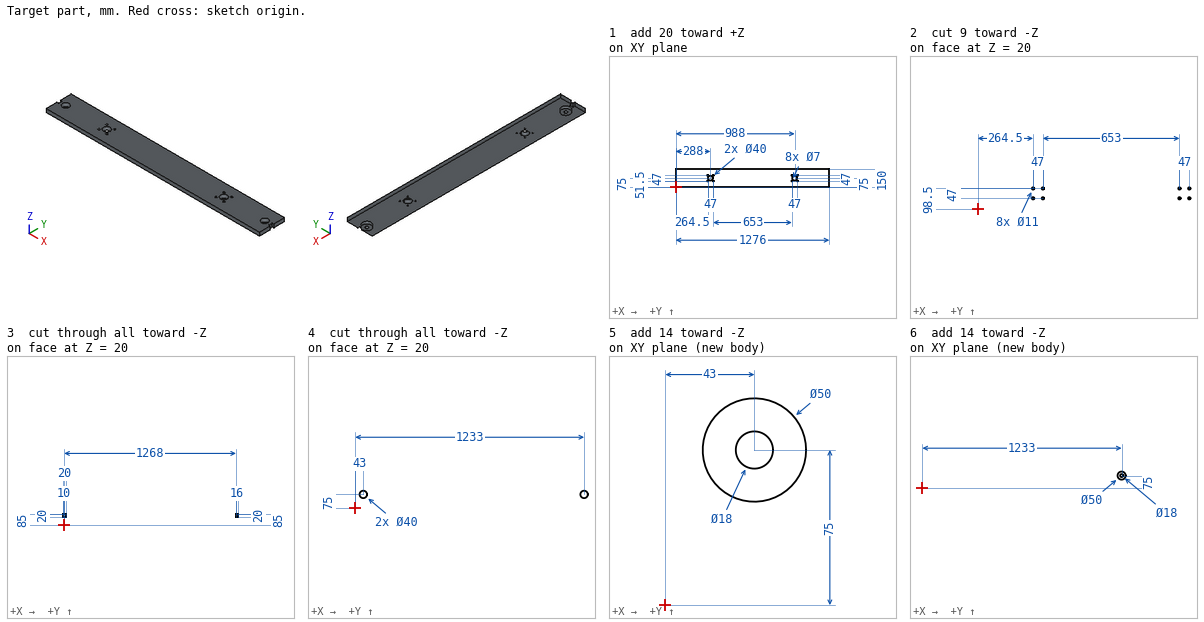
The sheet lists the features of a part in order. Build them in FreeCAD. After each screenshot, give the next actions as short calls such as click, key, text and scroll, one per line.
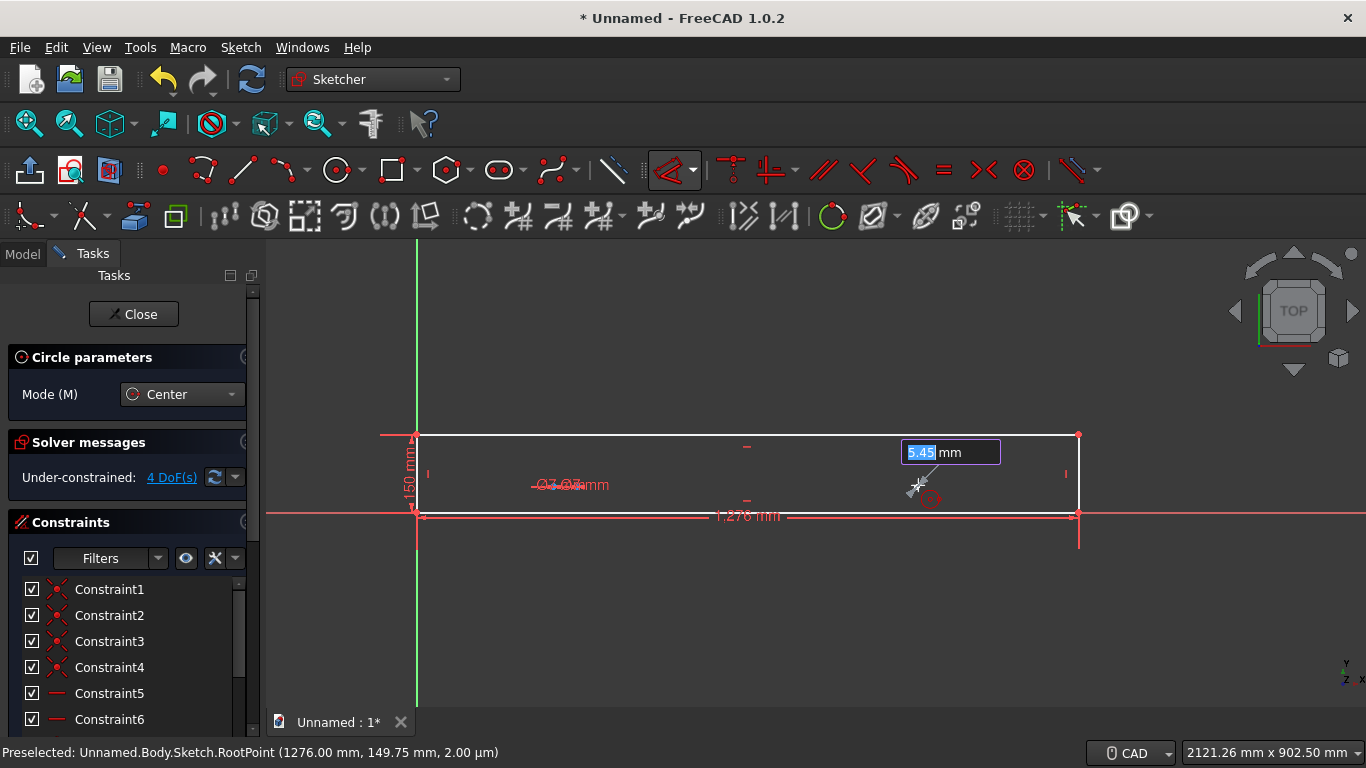
text(7)
key(Return)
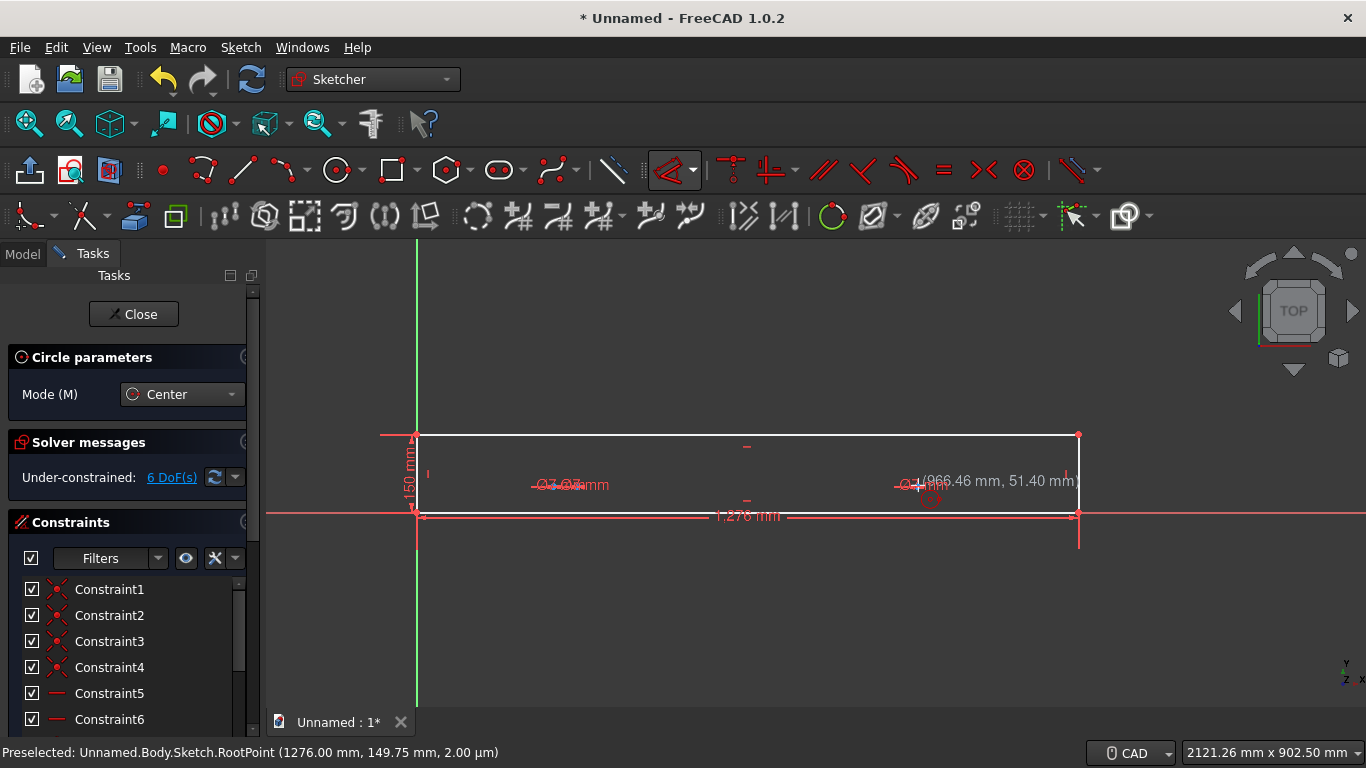
scroll(941, 486, up, 13)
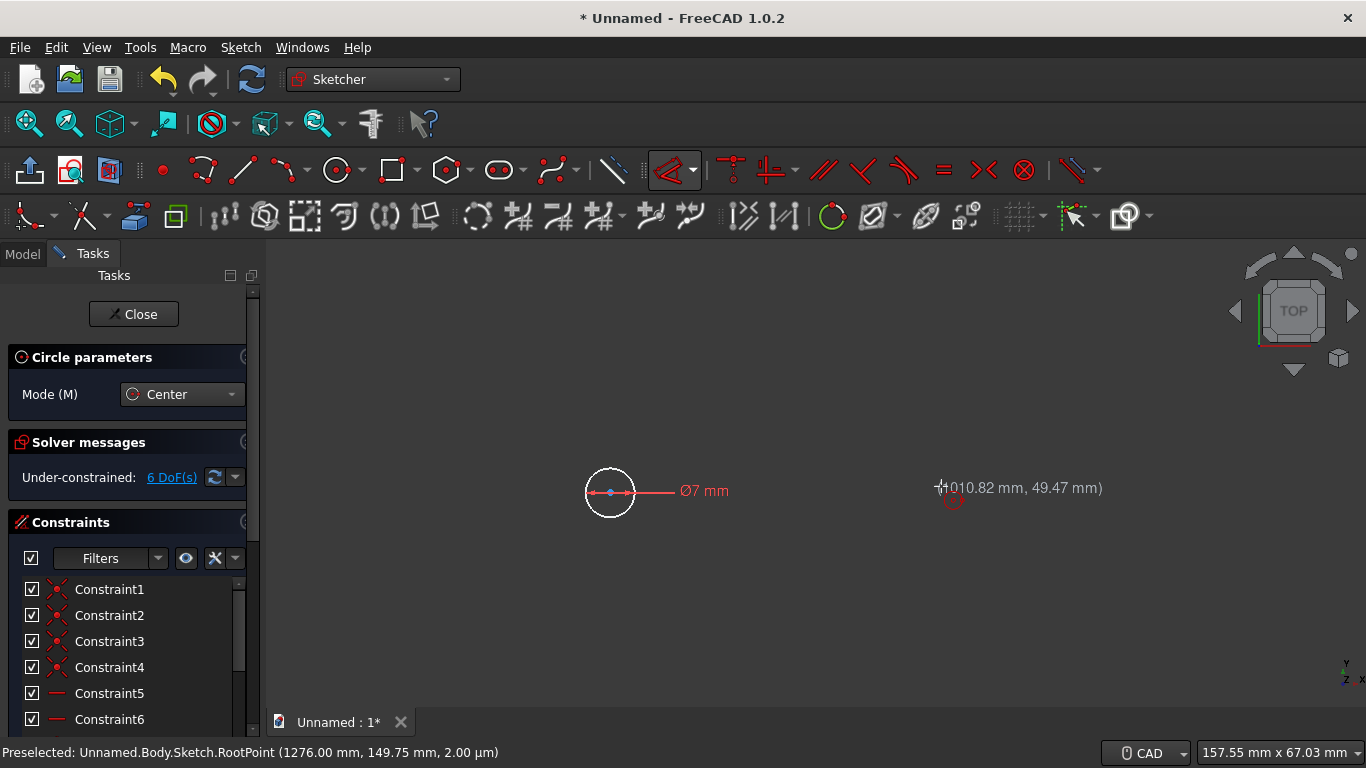
scroll(941, 486, down, 13)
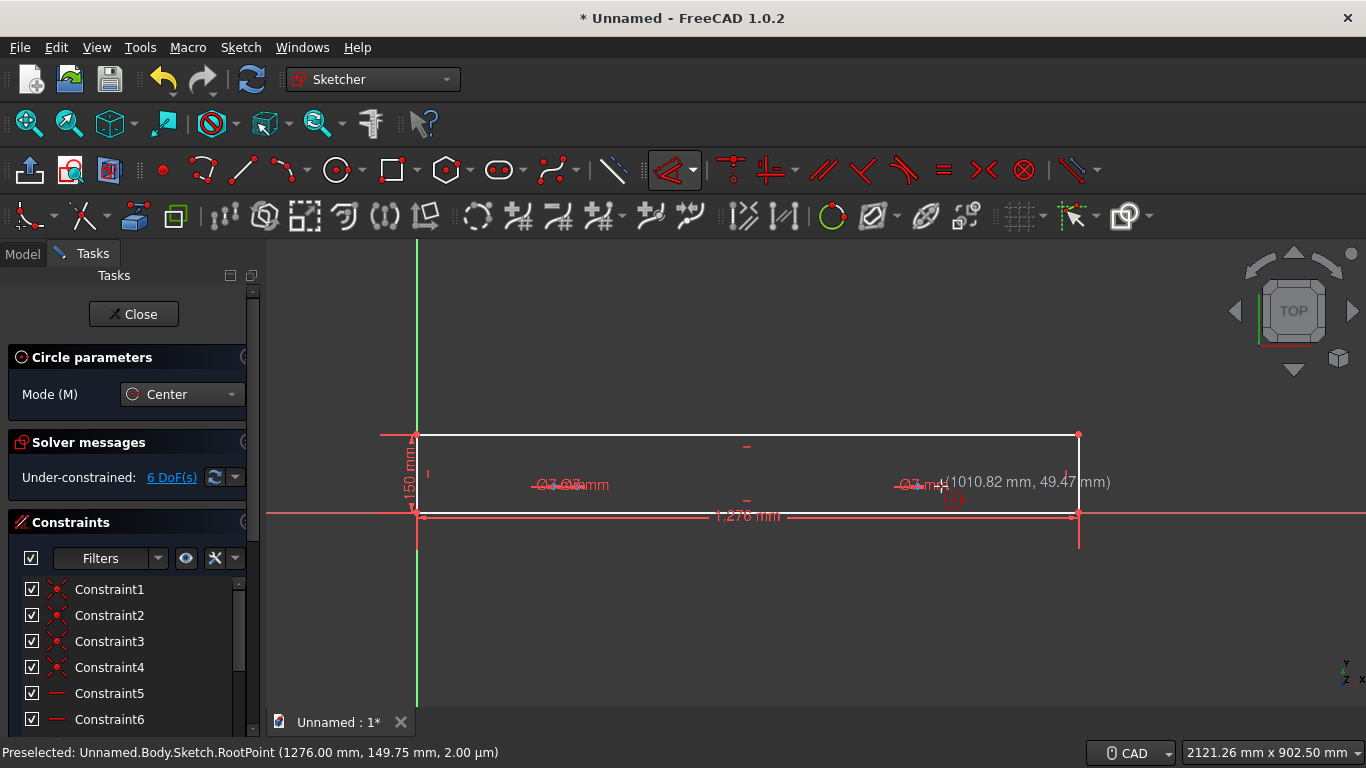
click(941, 486)
move(943, 485)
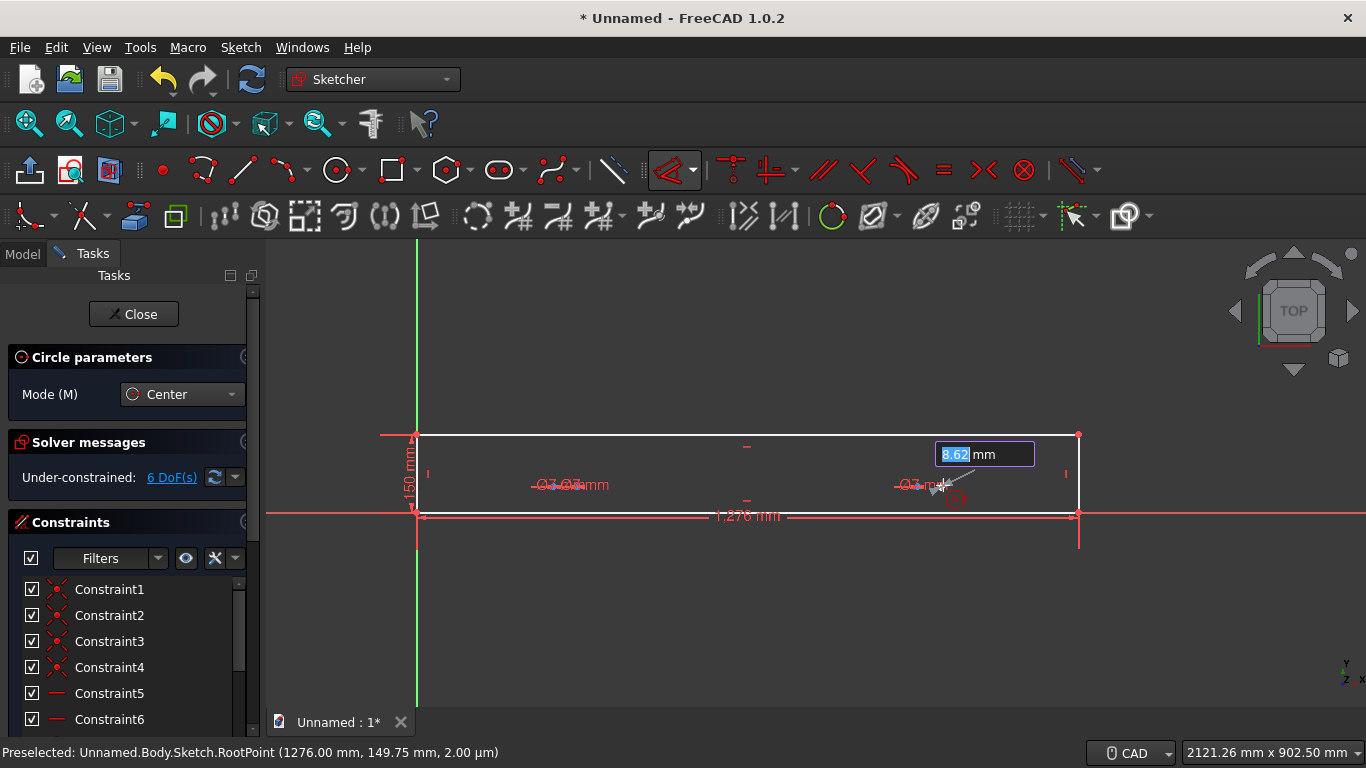
text(7)
key(Return)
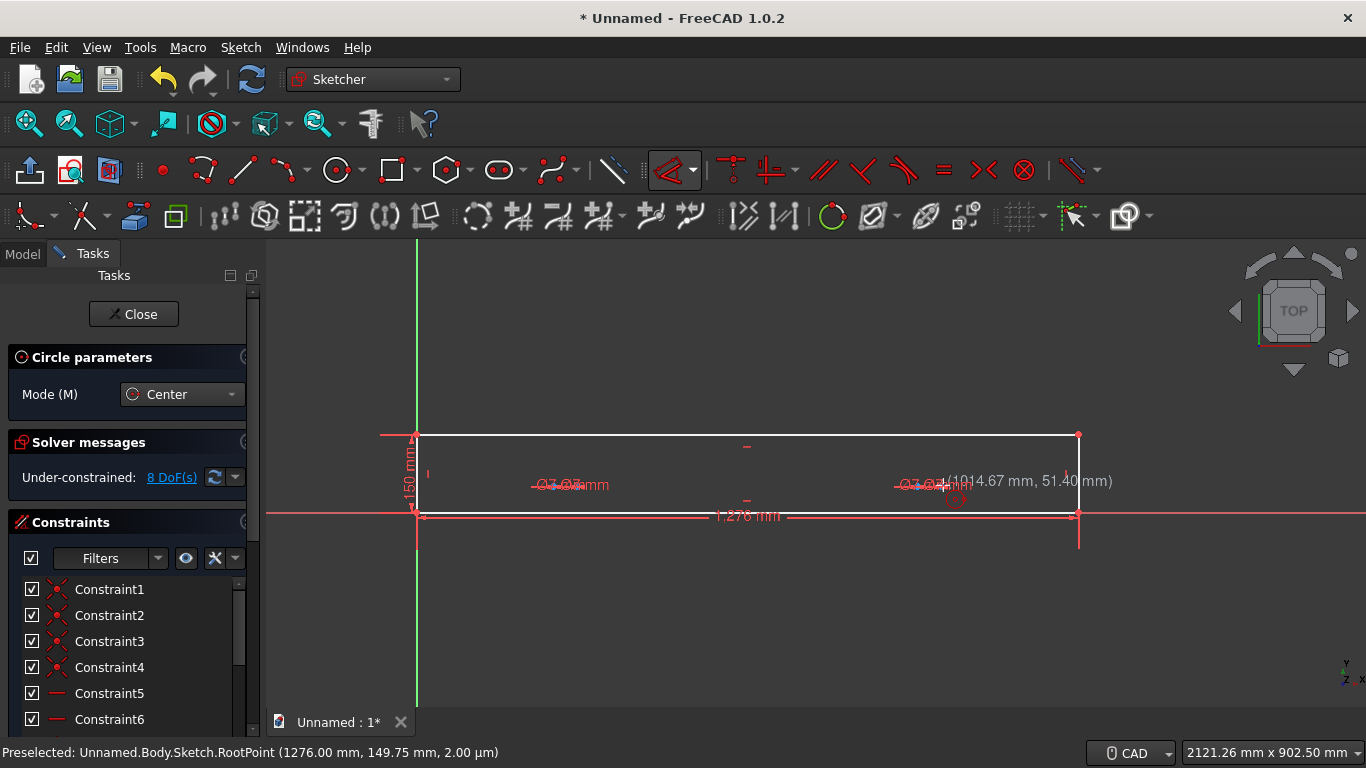
scroll(566, 474, up, 4)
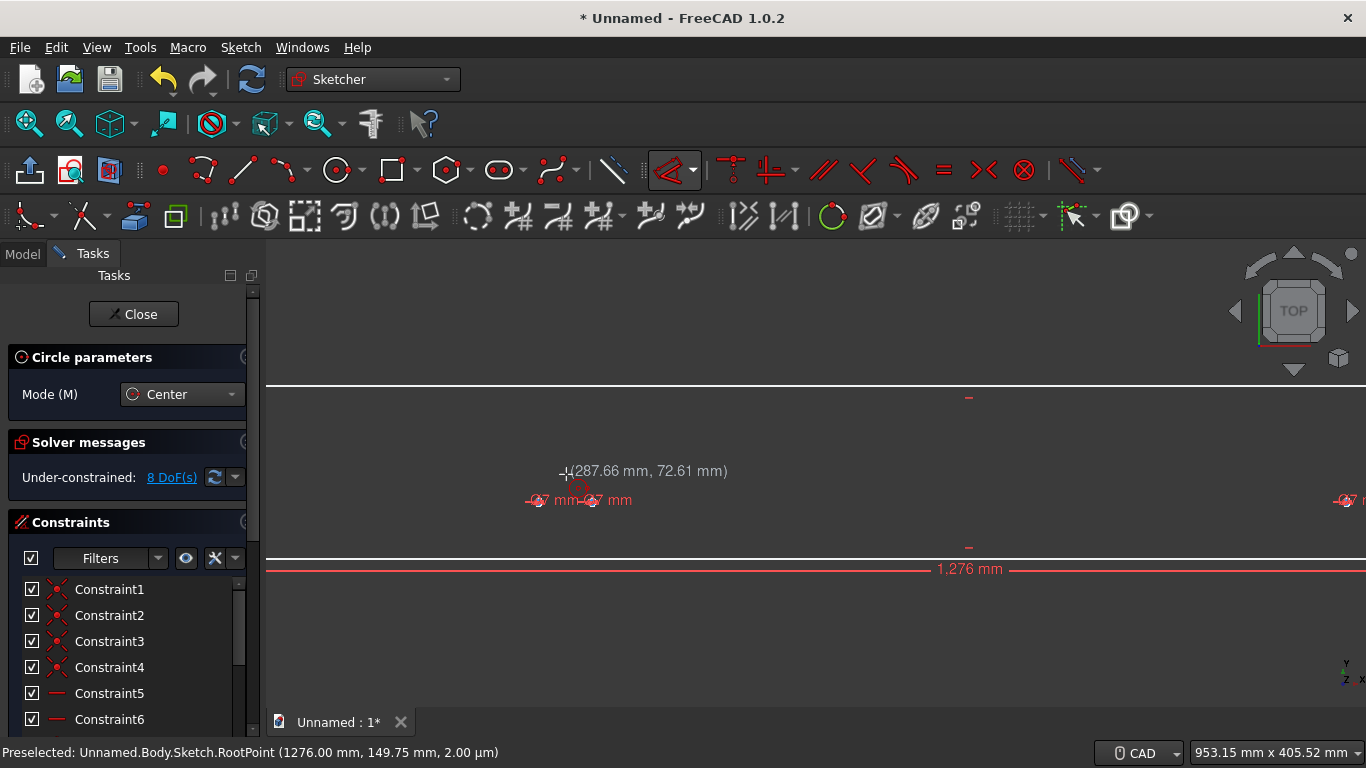
click(566, 473)
move(582, 457)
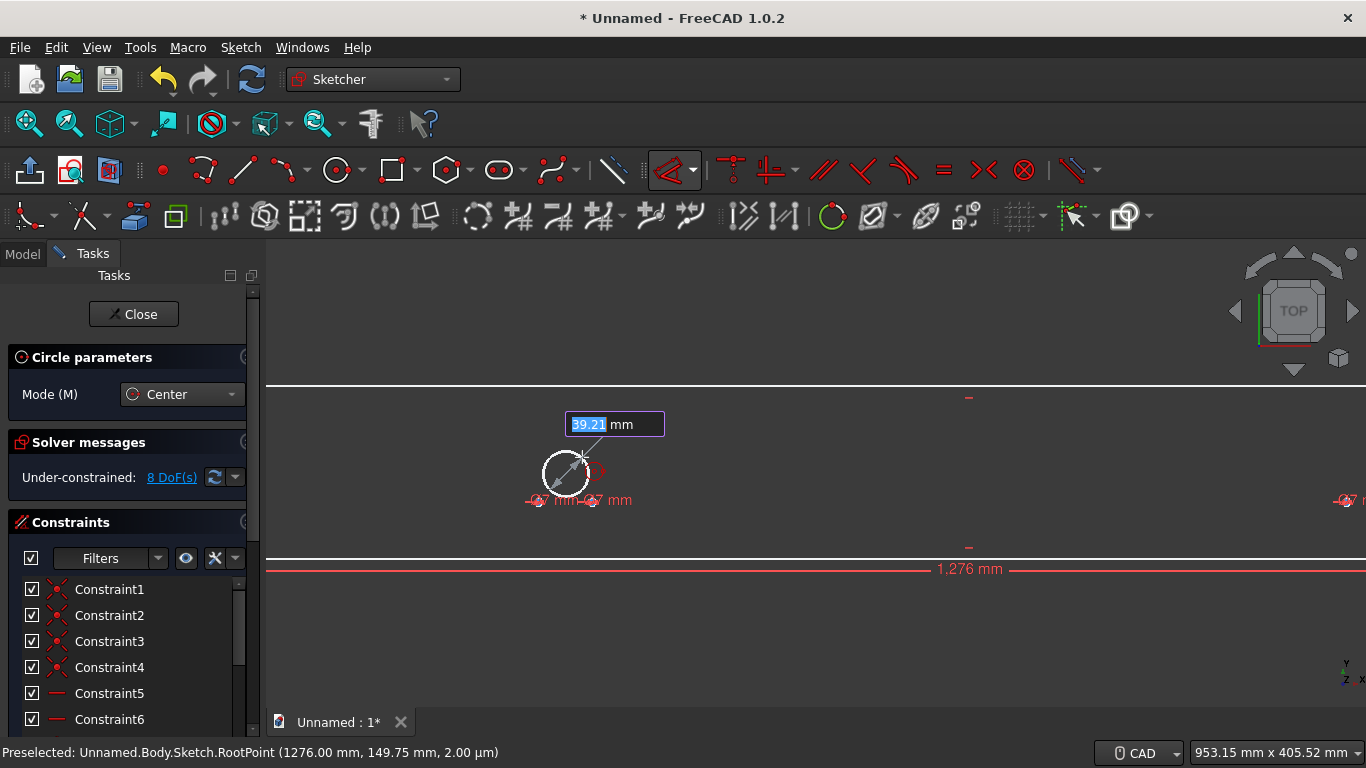
text(40)
key(Return)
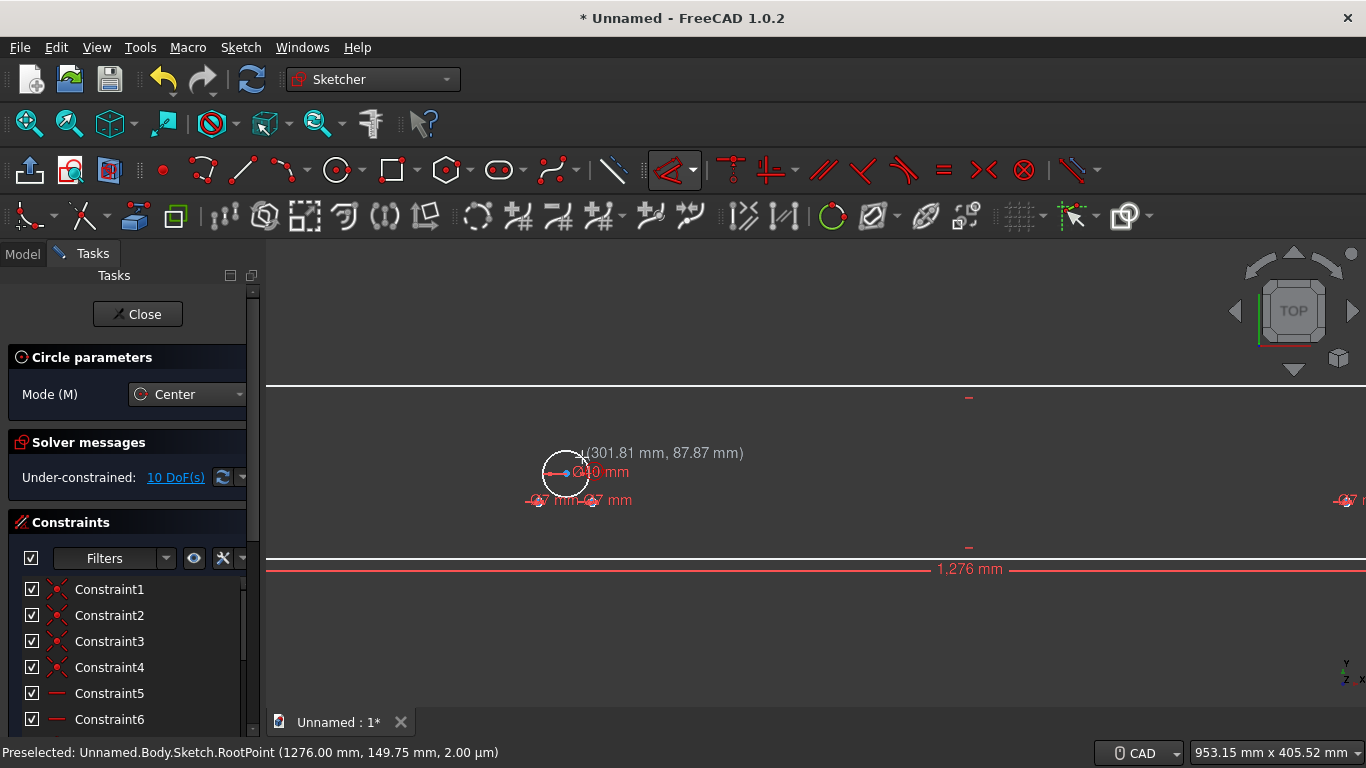
scroll(539, 446, up, 9)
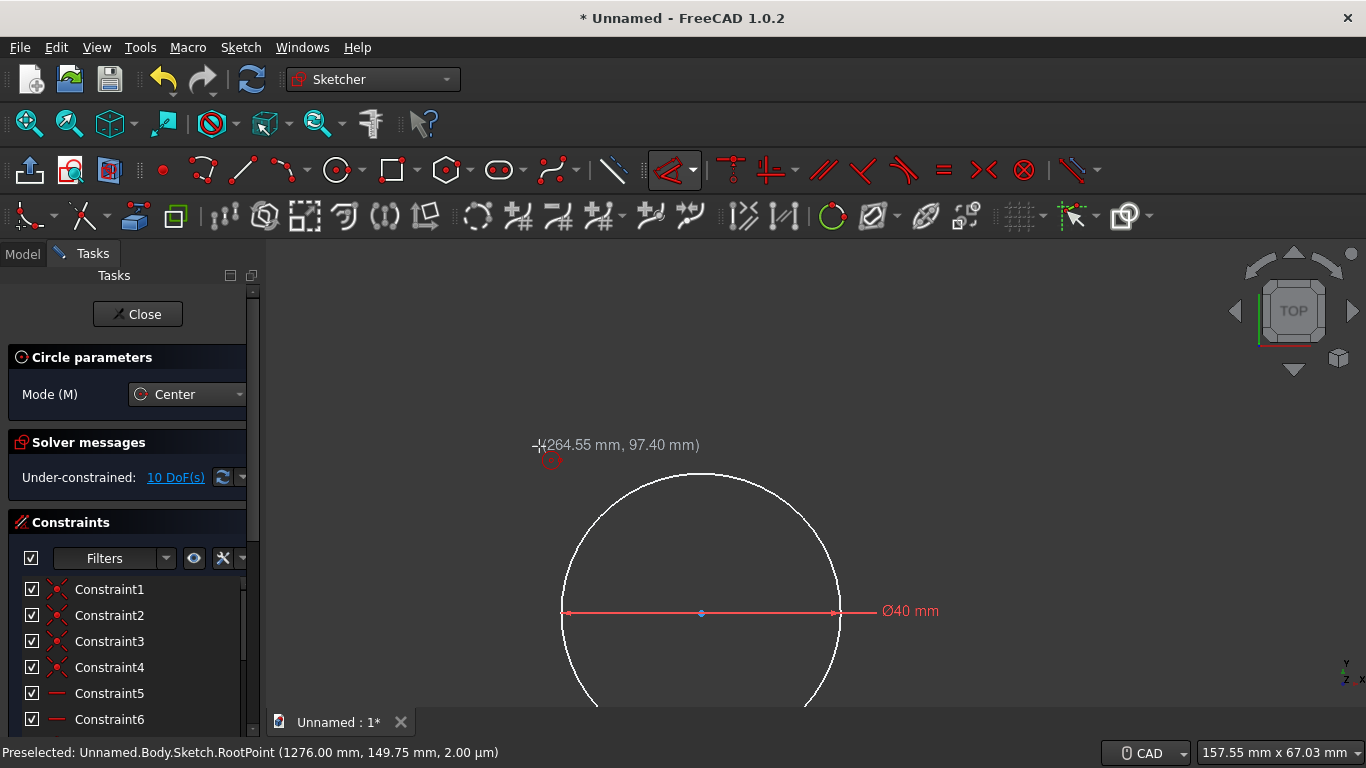
scroll(555, 462, down, 13)